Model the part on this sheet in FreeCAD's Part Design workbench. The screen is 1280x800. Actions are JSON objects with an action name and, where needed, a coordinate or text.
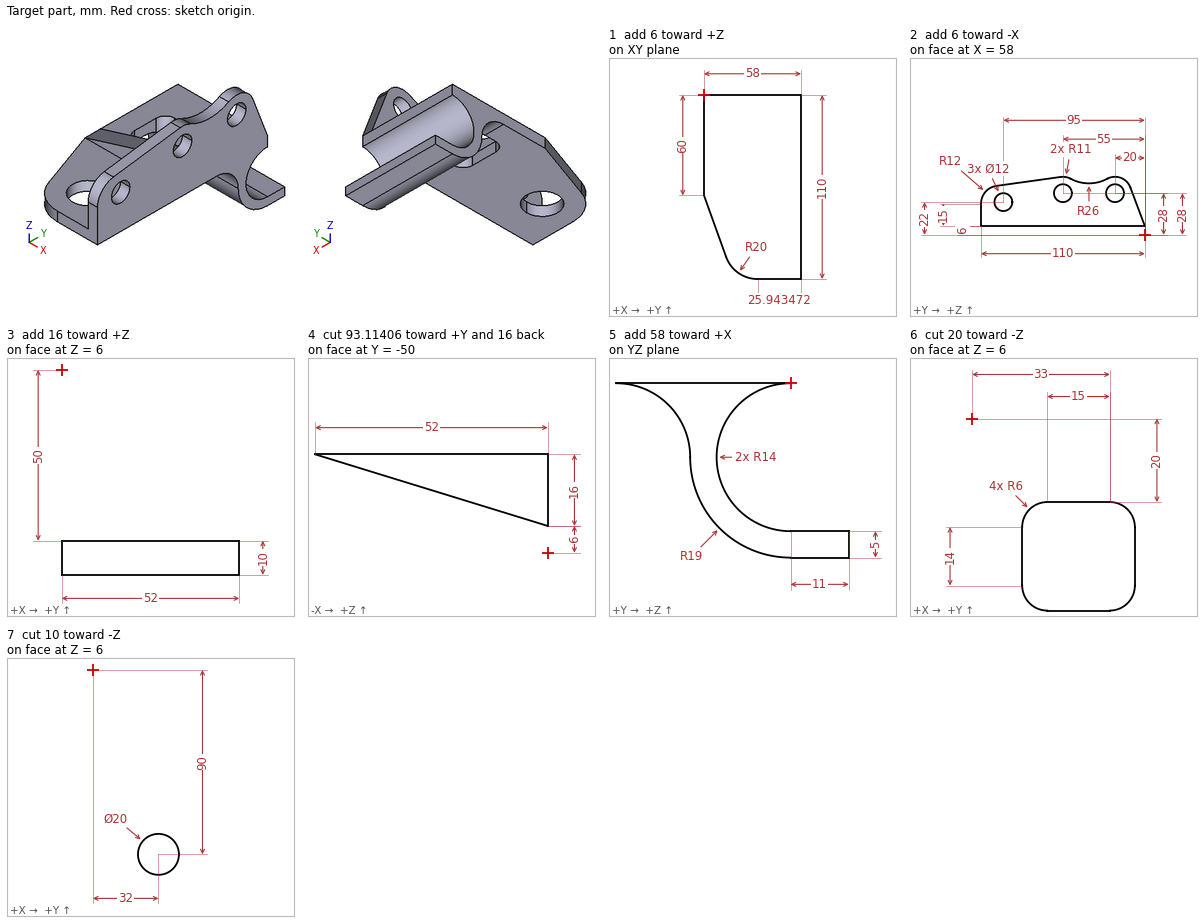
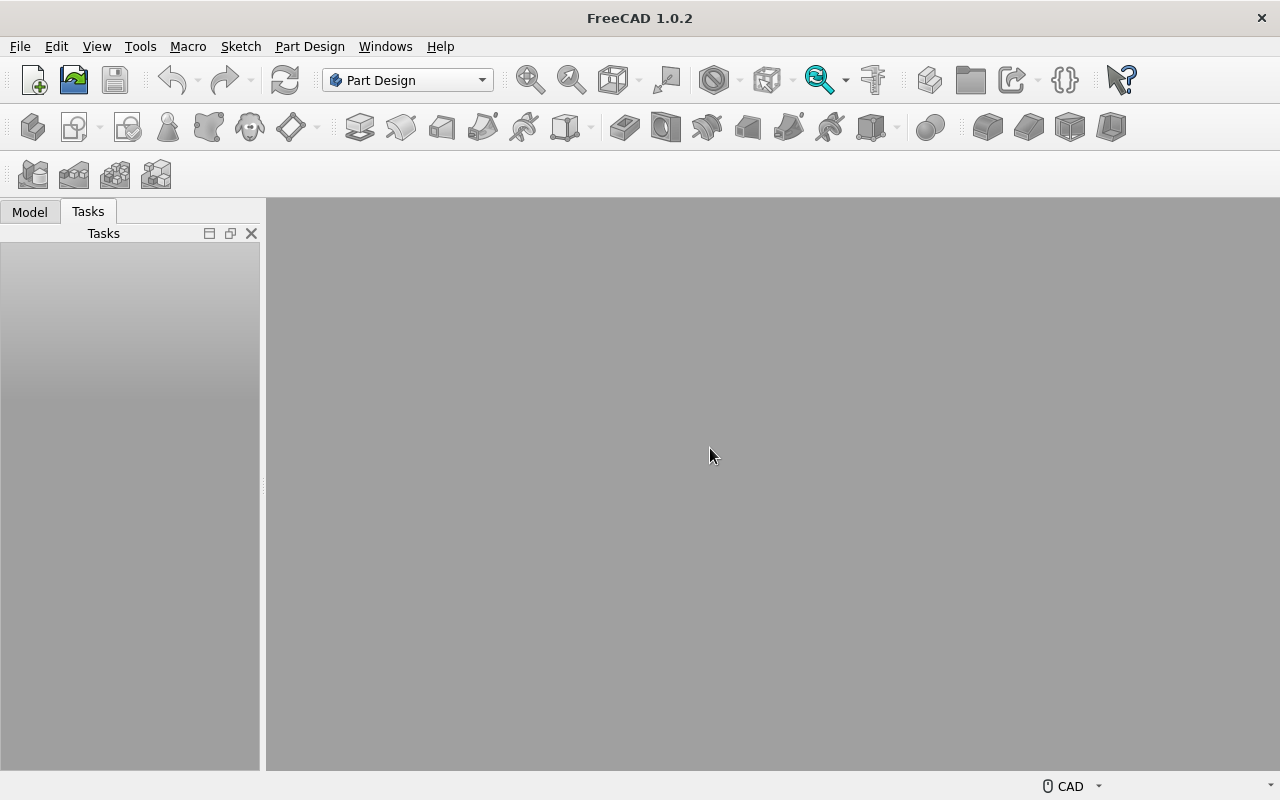
{"action": "left_click", "coordinate": [33, 80]}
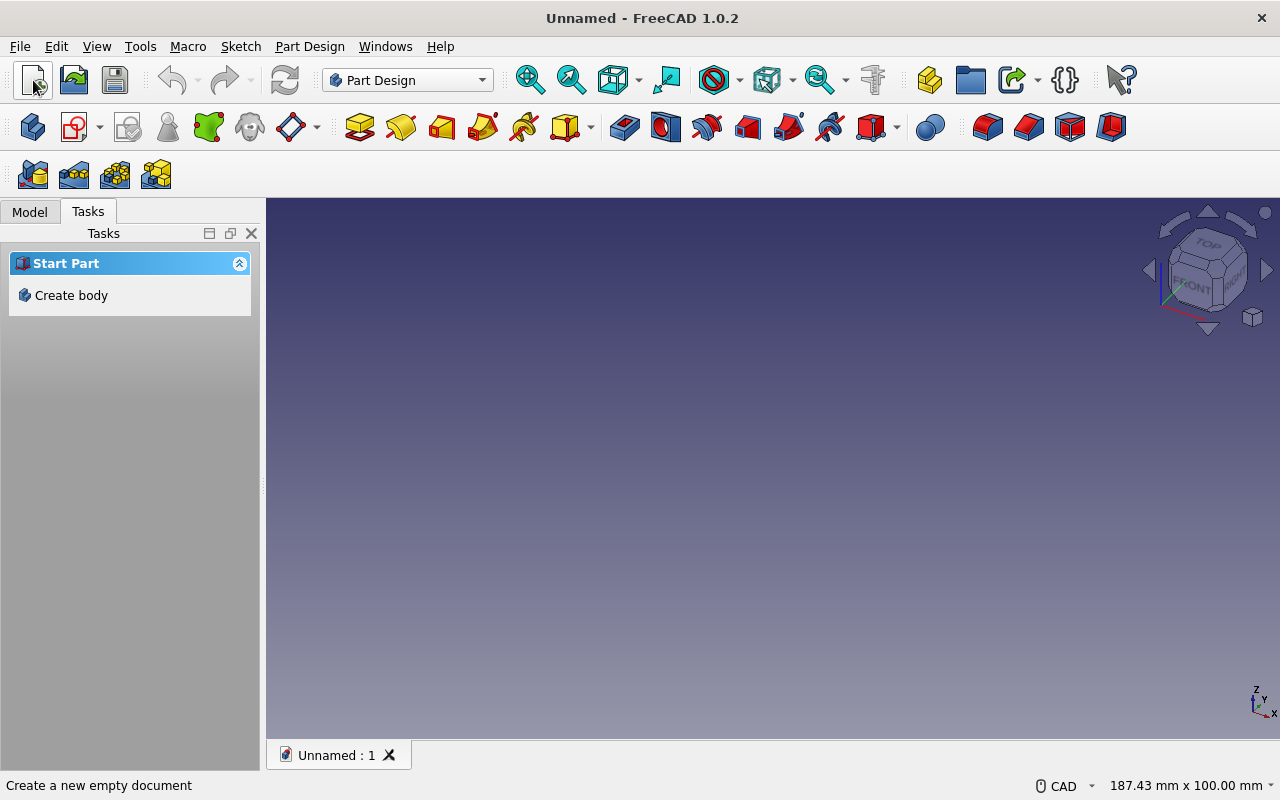
{"action": "left_click", "coordinate": [74, 128]}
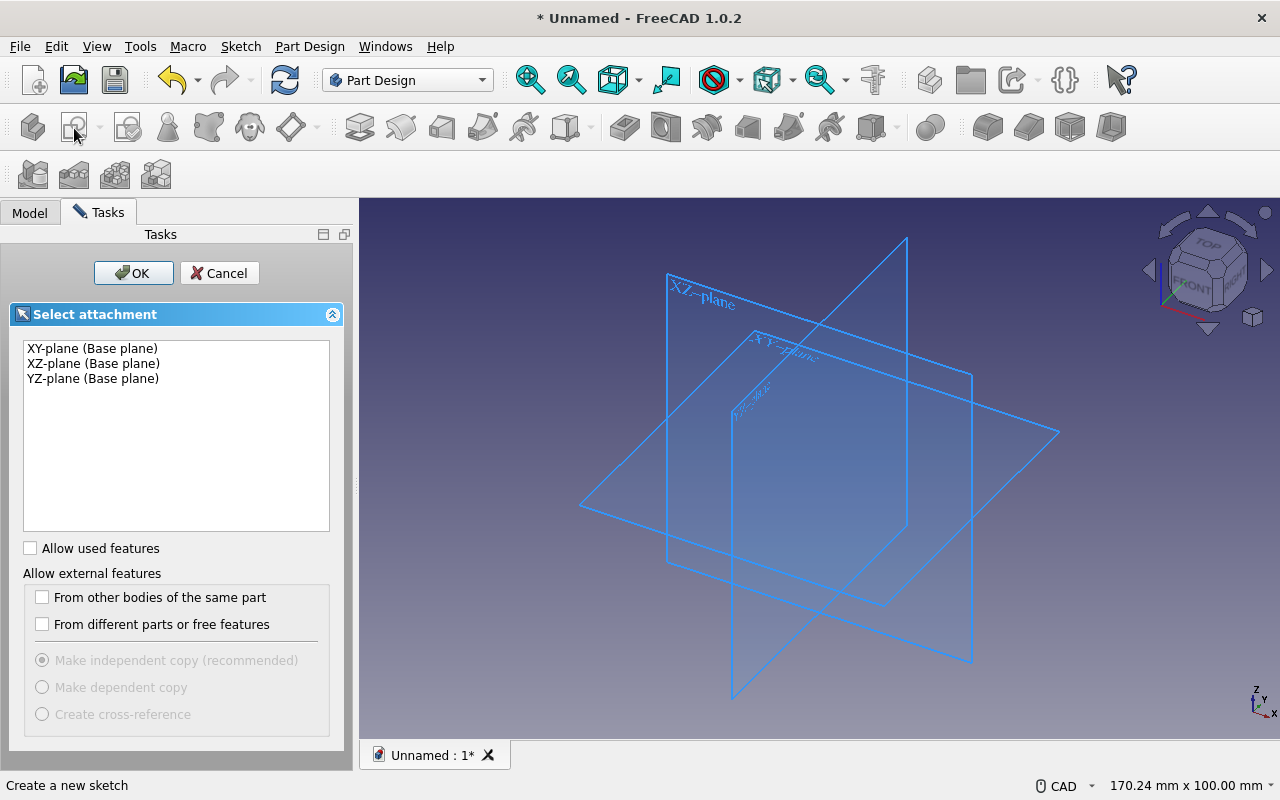
{"action": "left_click", "coordinate": [84, 348]}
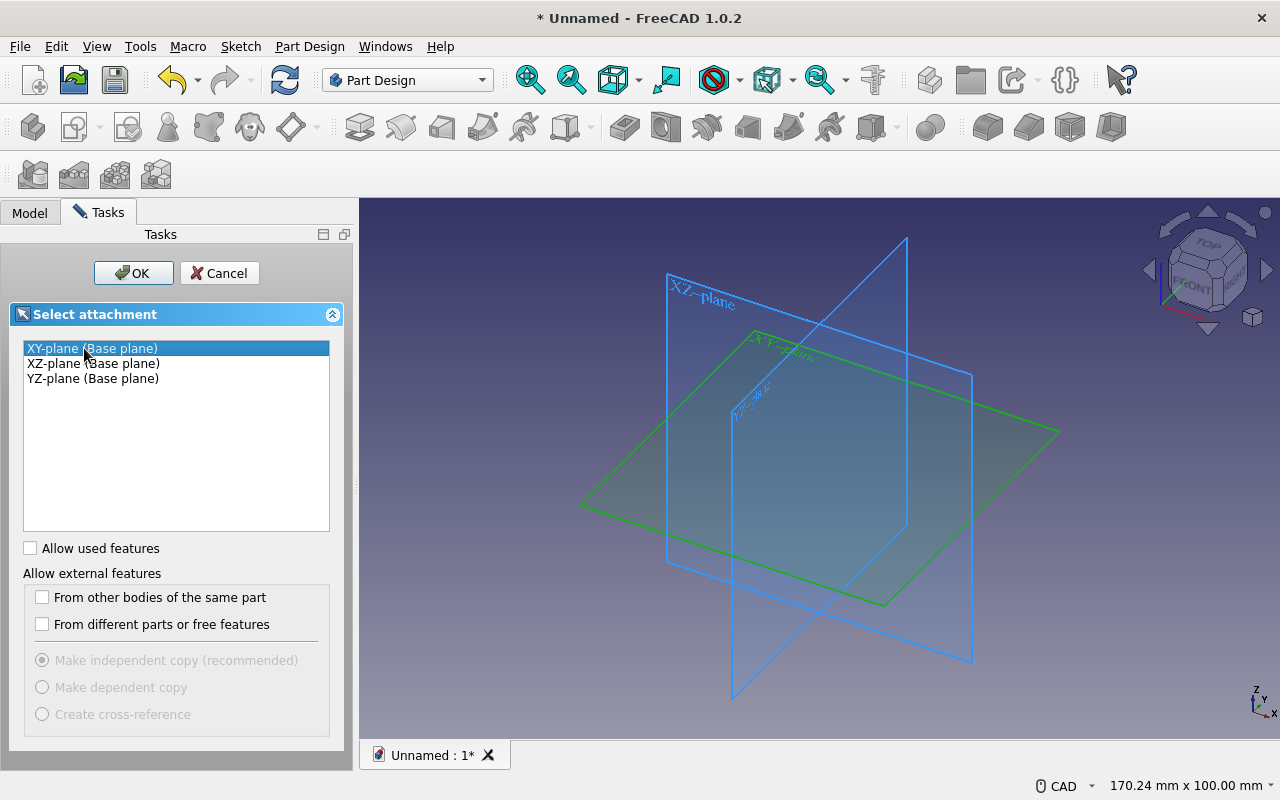
{"action": "left_click", "coordinate": [134, 273]}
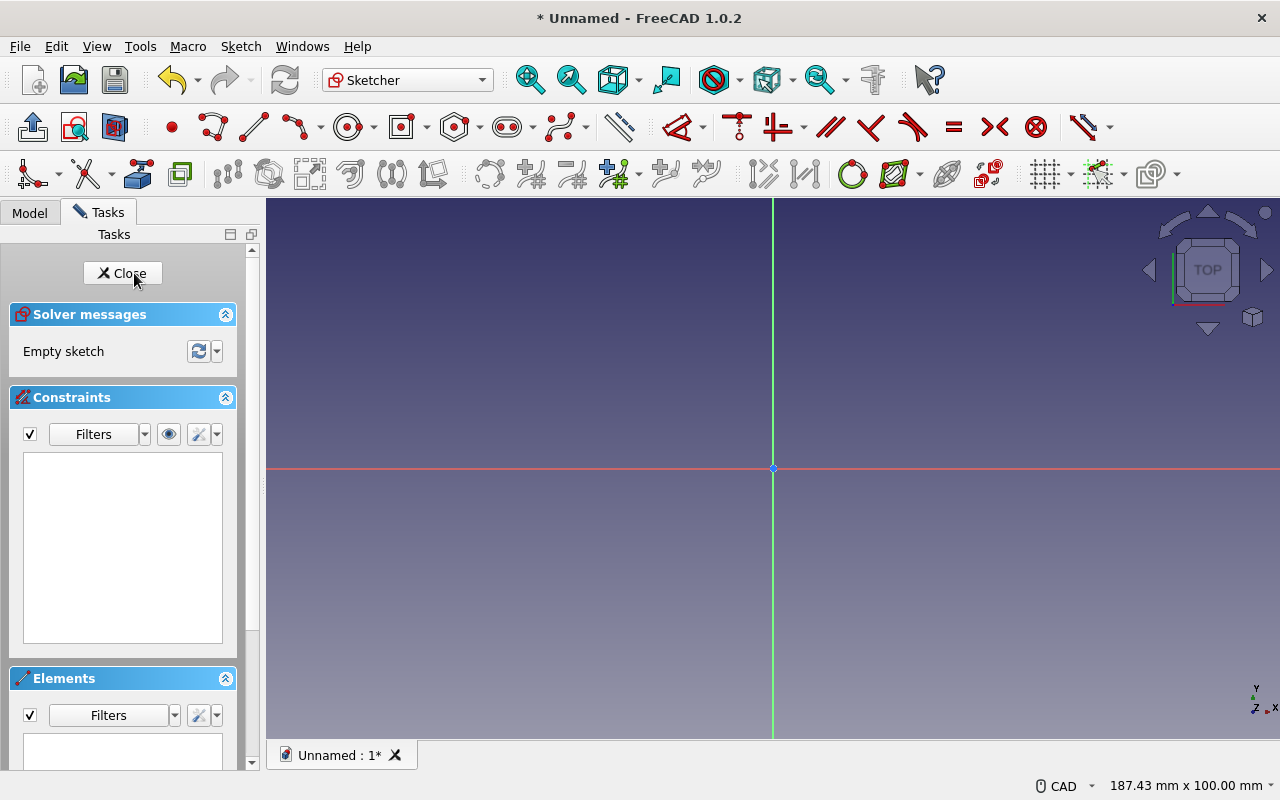
{"action": "scroll", "coordinate": [430, 226], "scroll_direction": "down", "scroll_amount": 3}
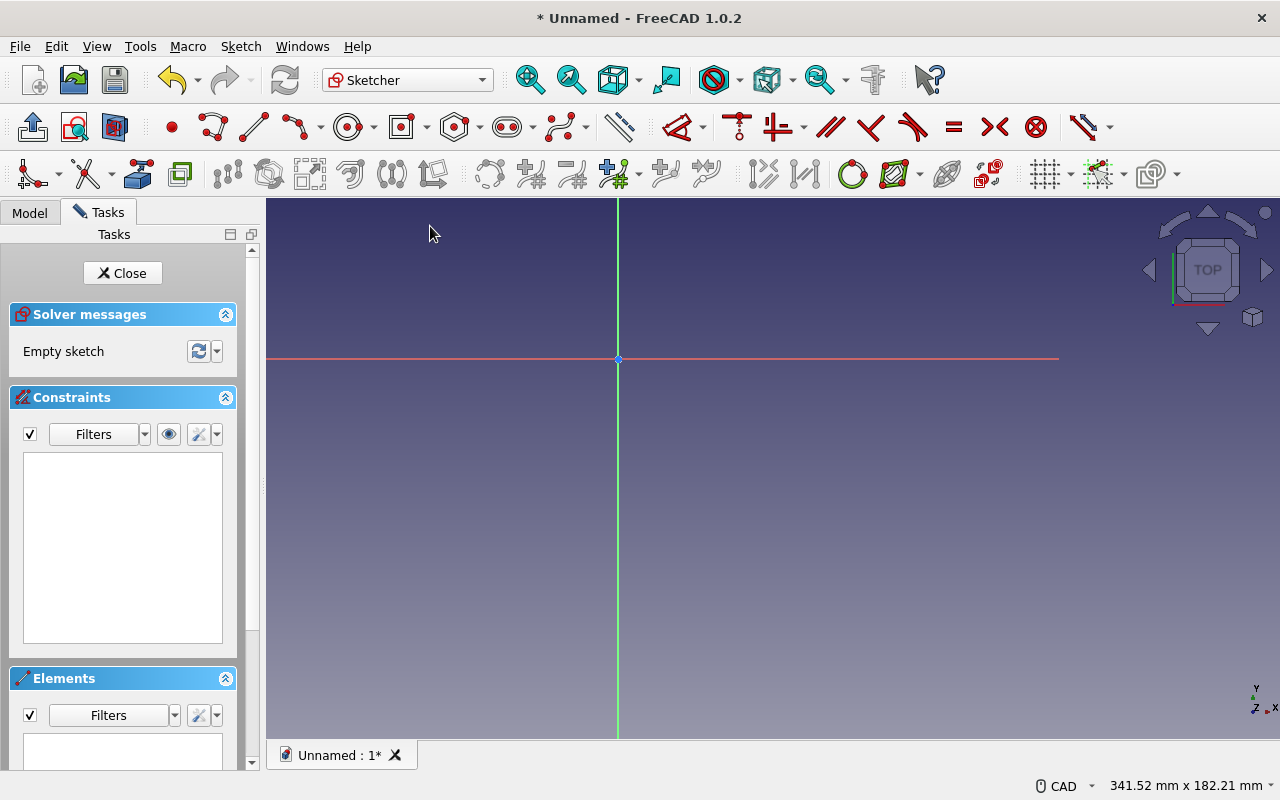
{"action": "left_click", "coordinate": [213, 128]}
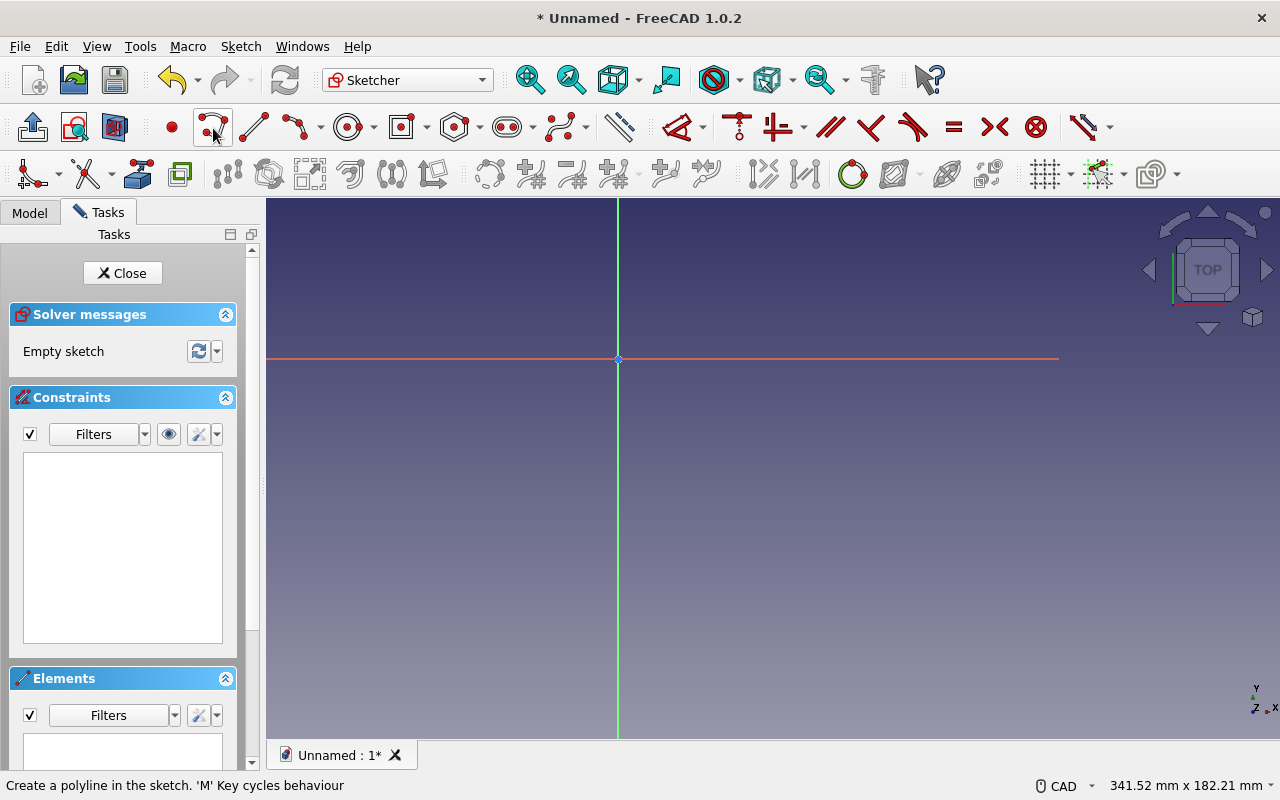
{"action": "left_click", "coordinate": [713, 686]}
{"action": "left_click", "coordinate": [791, 686]}
{"action": "left_click", "coordinate": [791, 359]}
{"action": "left_click", "coordinate": [618, 359]}
{"action": "left_click", "coordinate": [627, 537]}
{"action": "left_click", "coordinate": [658, 646]}
{"action": "right_click", "coordinate": [658, 646]}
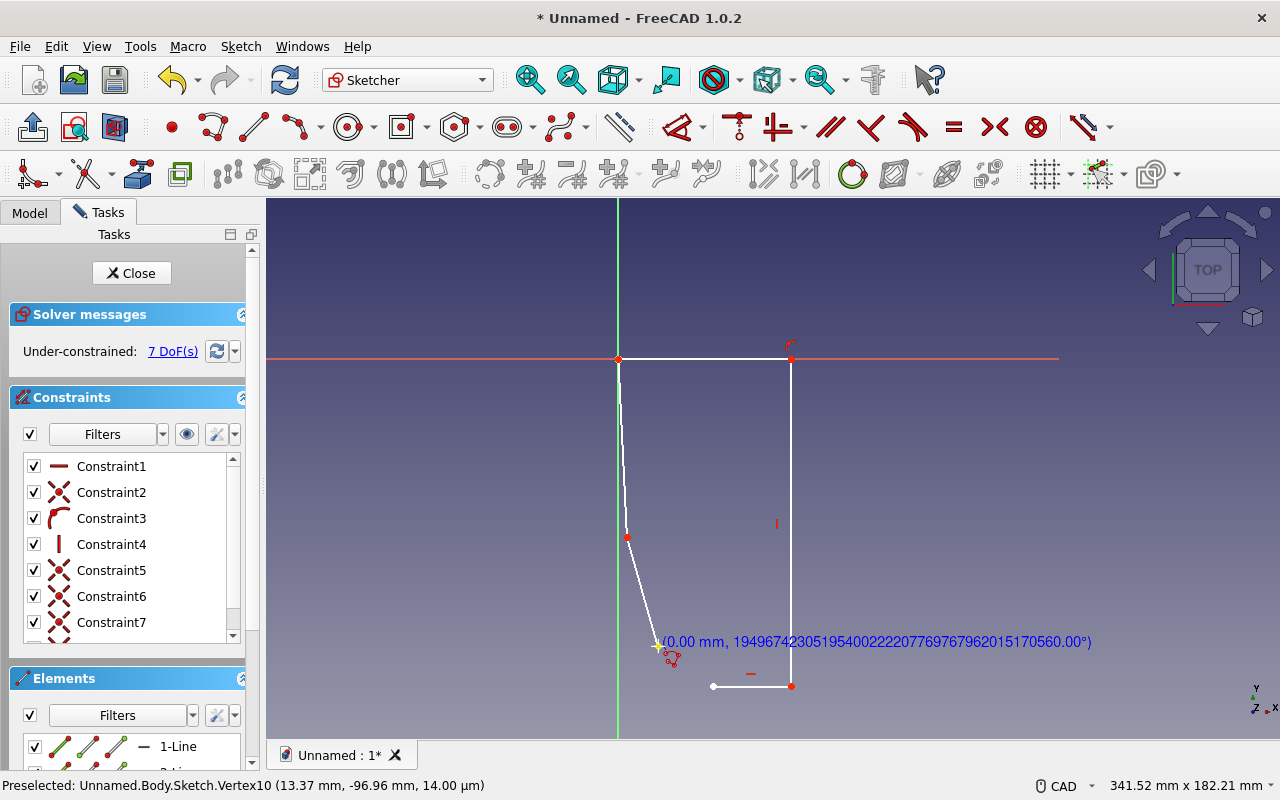
{"action": "left_click", "coordinate": [294, 128]}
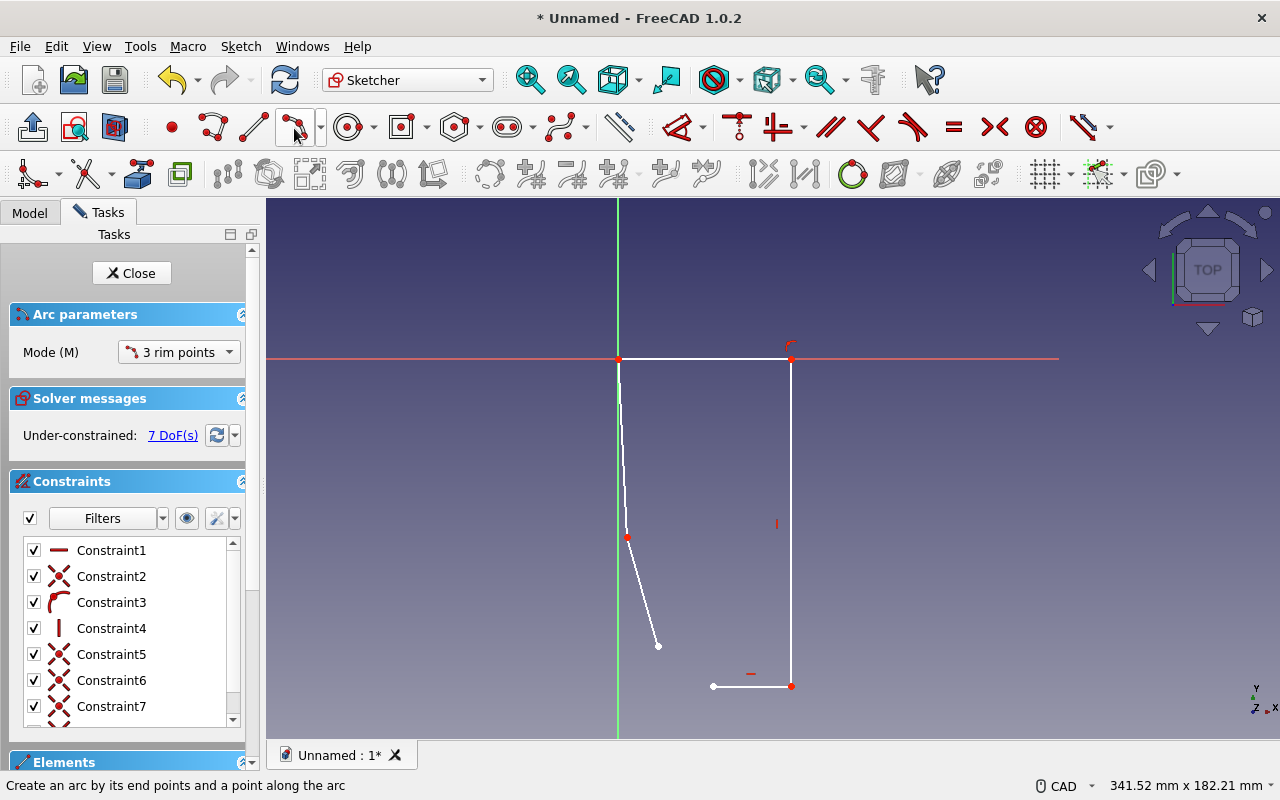
{"action": "left_click", "coordinate": [658, 647]}
{"action": "left_click", "coordinate": [713, 687]}